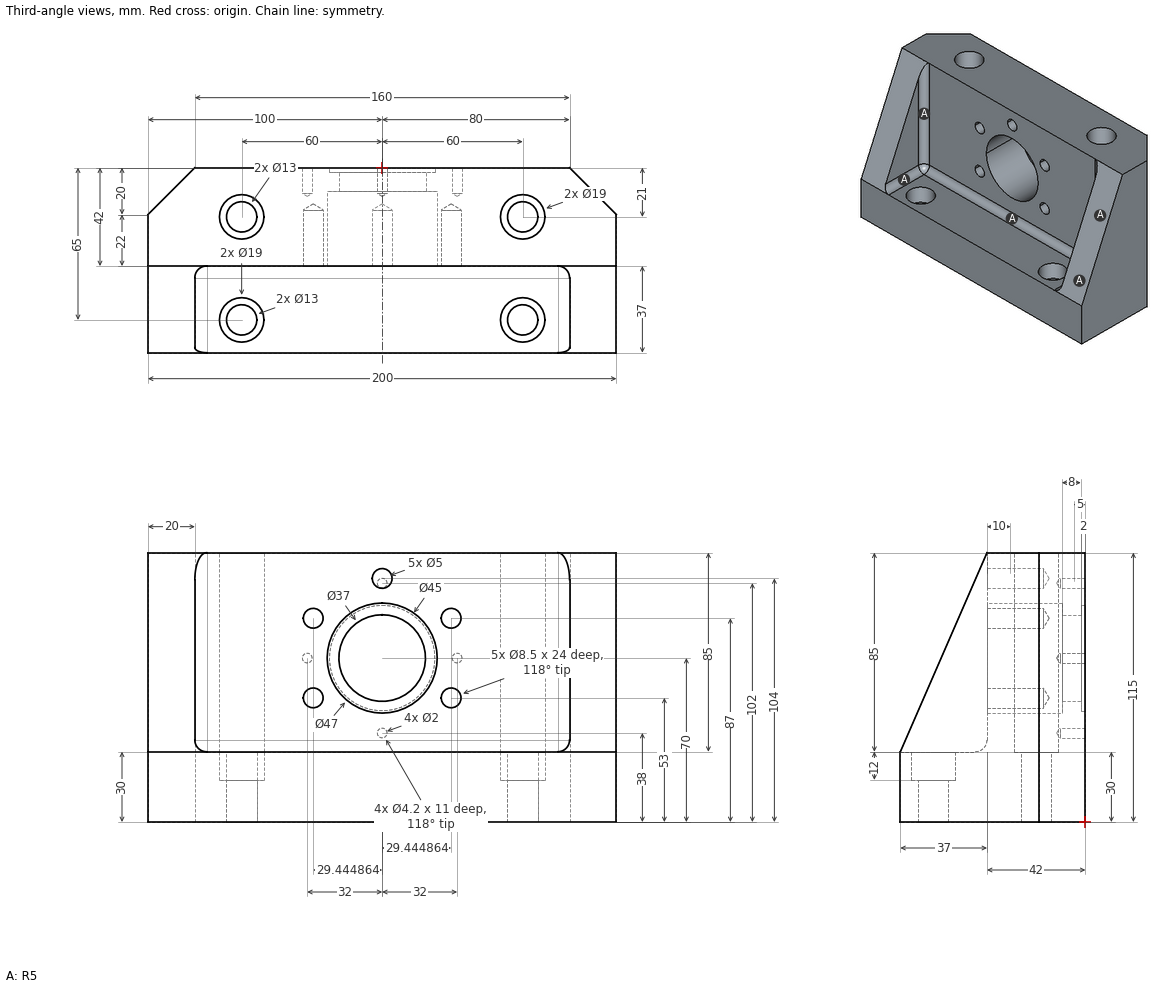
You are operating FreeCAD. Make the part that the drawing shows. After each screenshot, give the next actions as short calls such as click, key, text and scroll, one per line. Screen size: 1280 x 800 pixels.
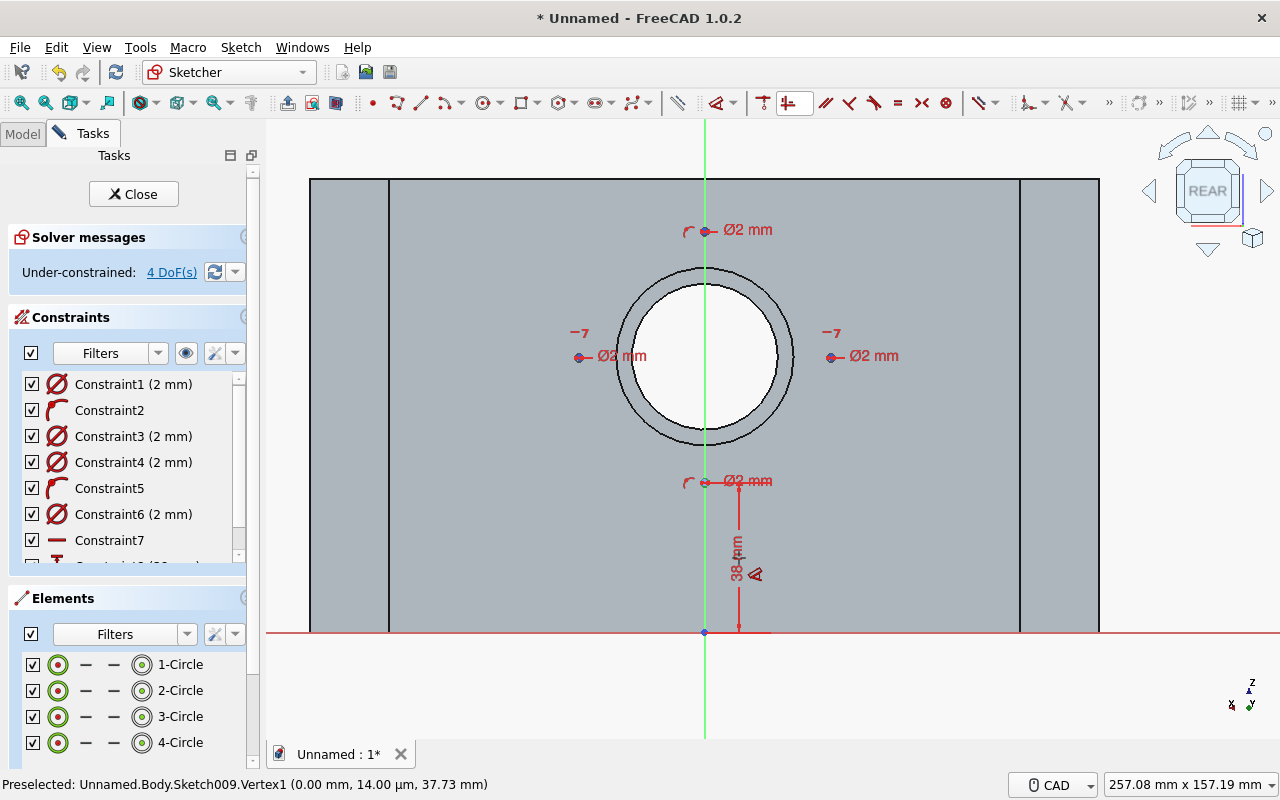
click(579, 358)
click(642, 667)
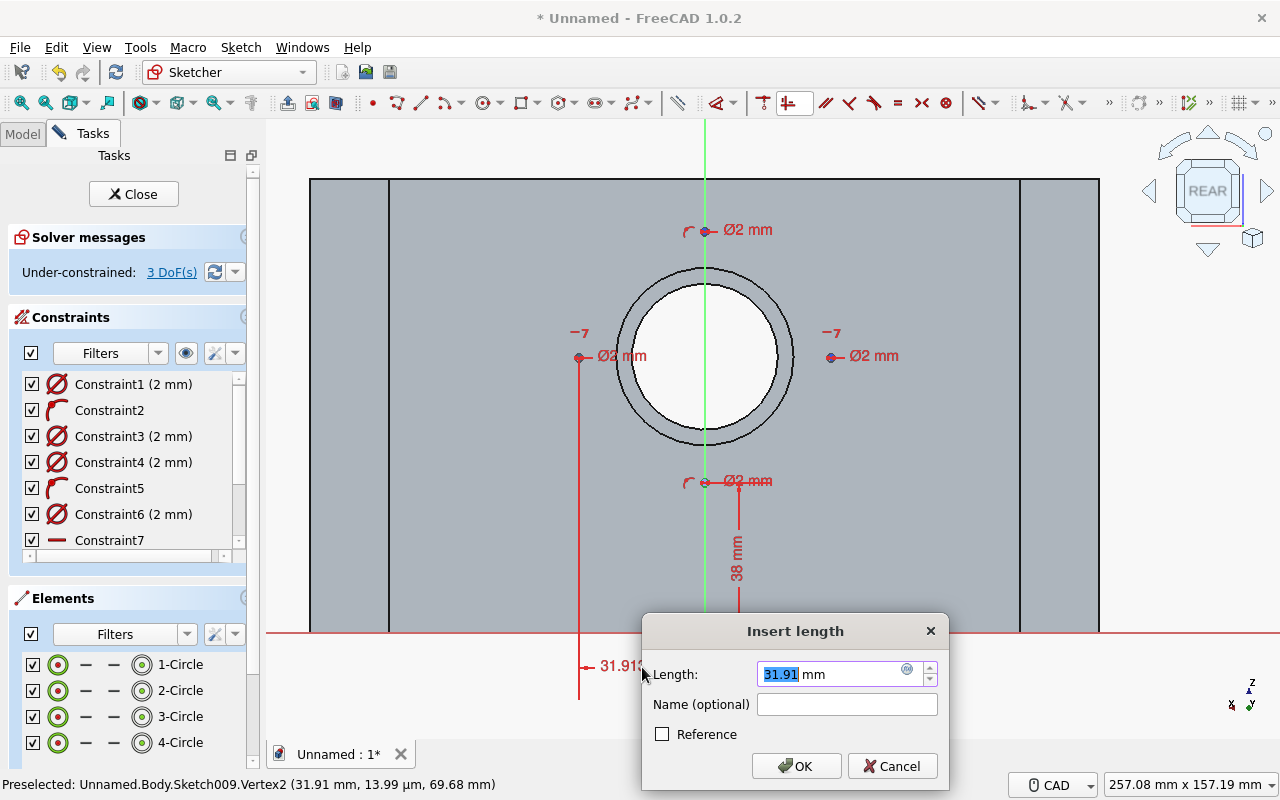
text(32)
key(Return)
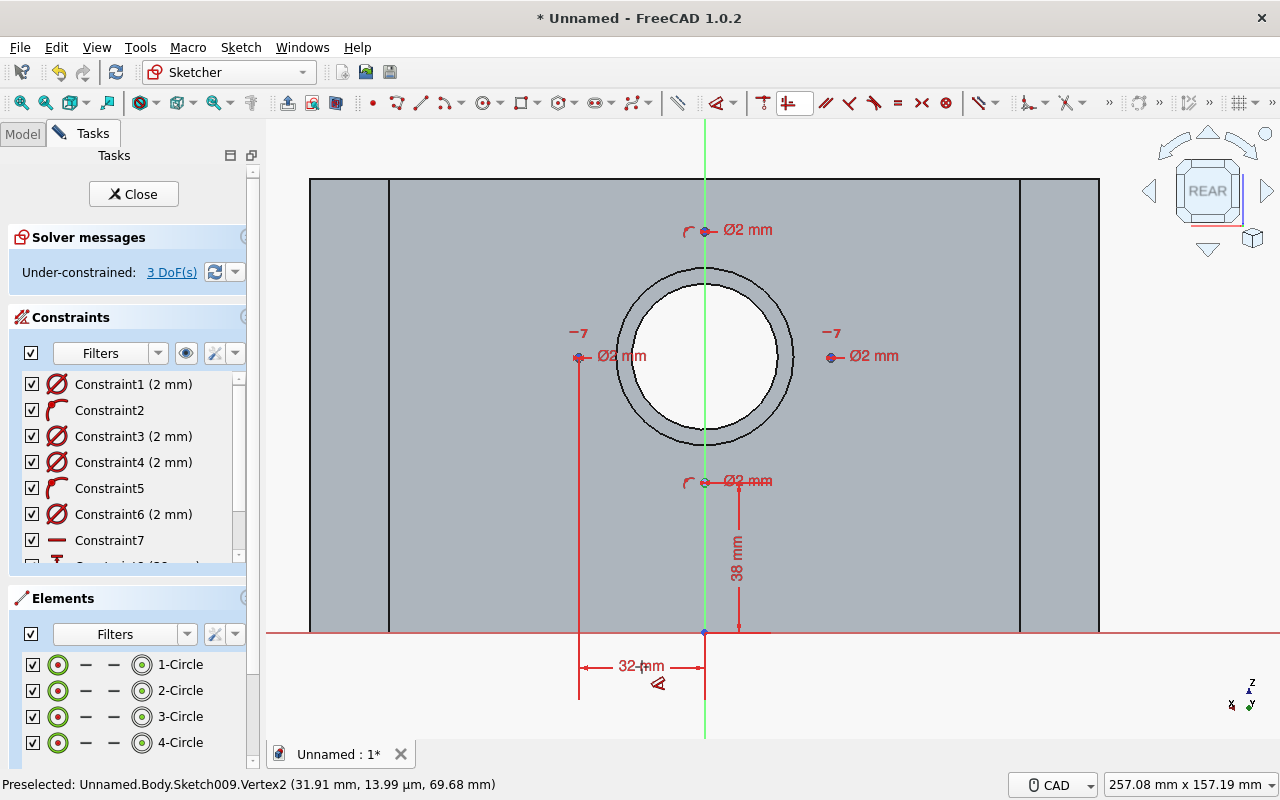
click(579, 358)
click(545, 495)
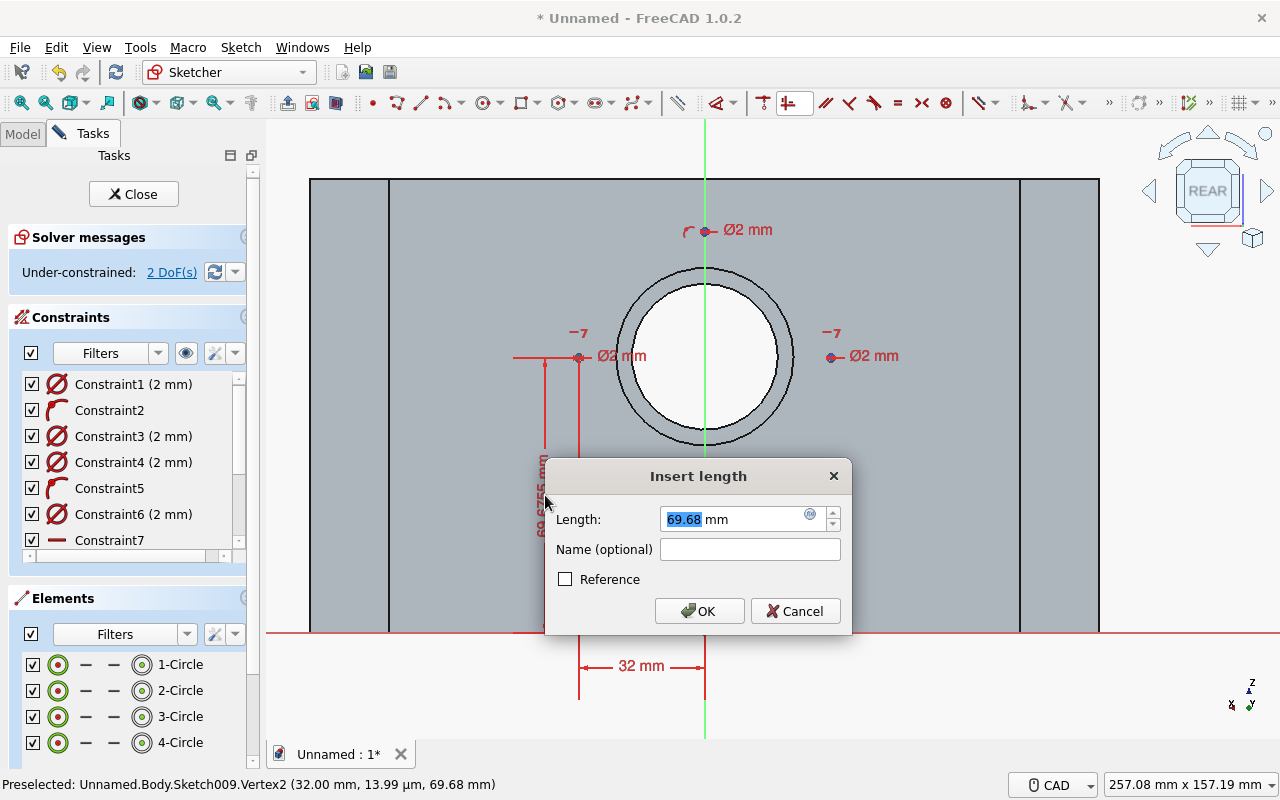
text(70)
key(Return)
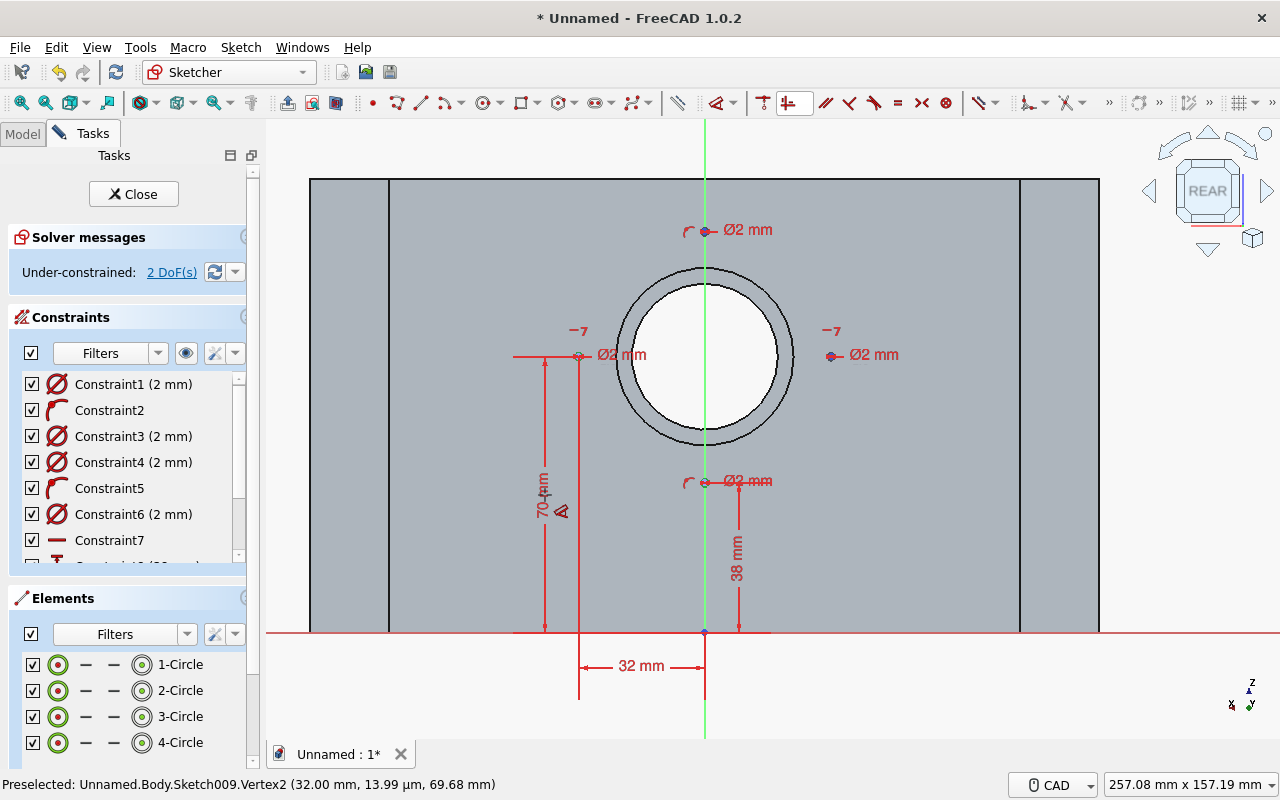
click(831, 357)
click(768, 667)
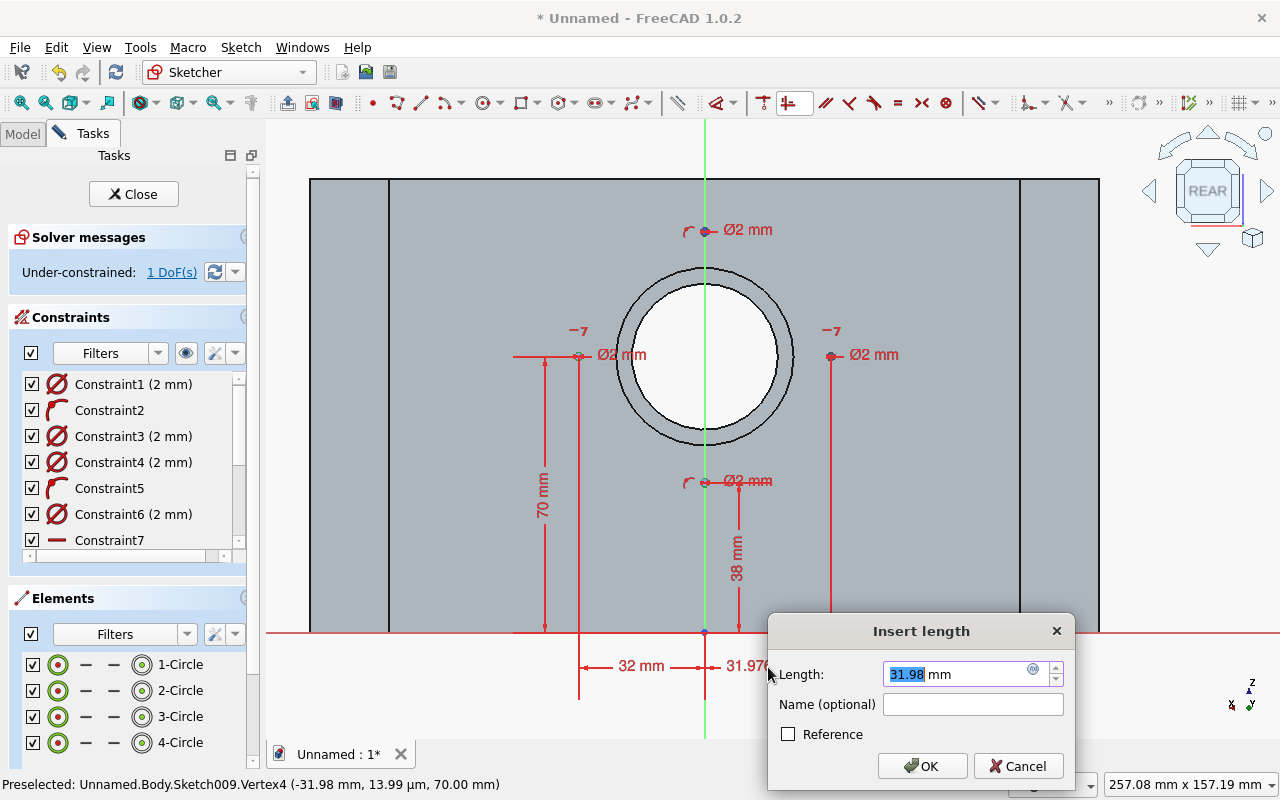
text(32)
key(Return)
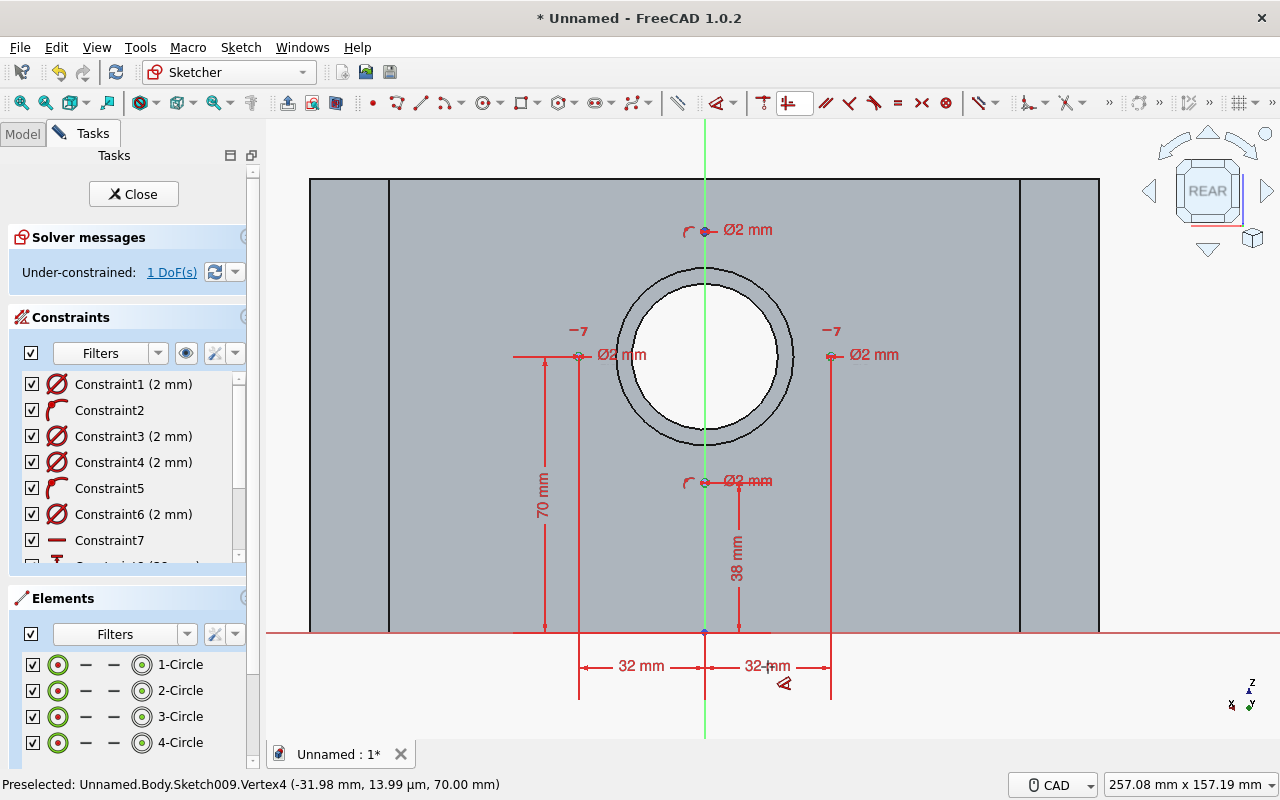
click(705, 232)
click(739, 432)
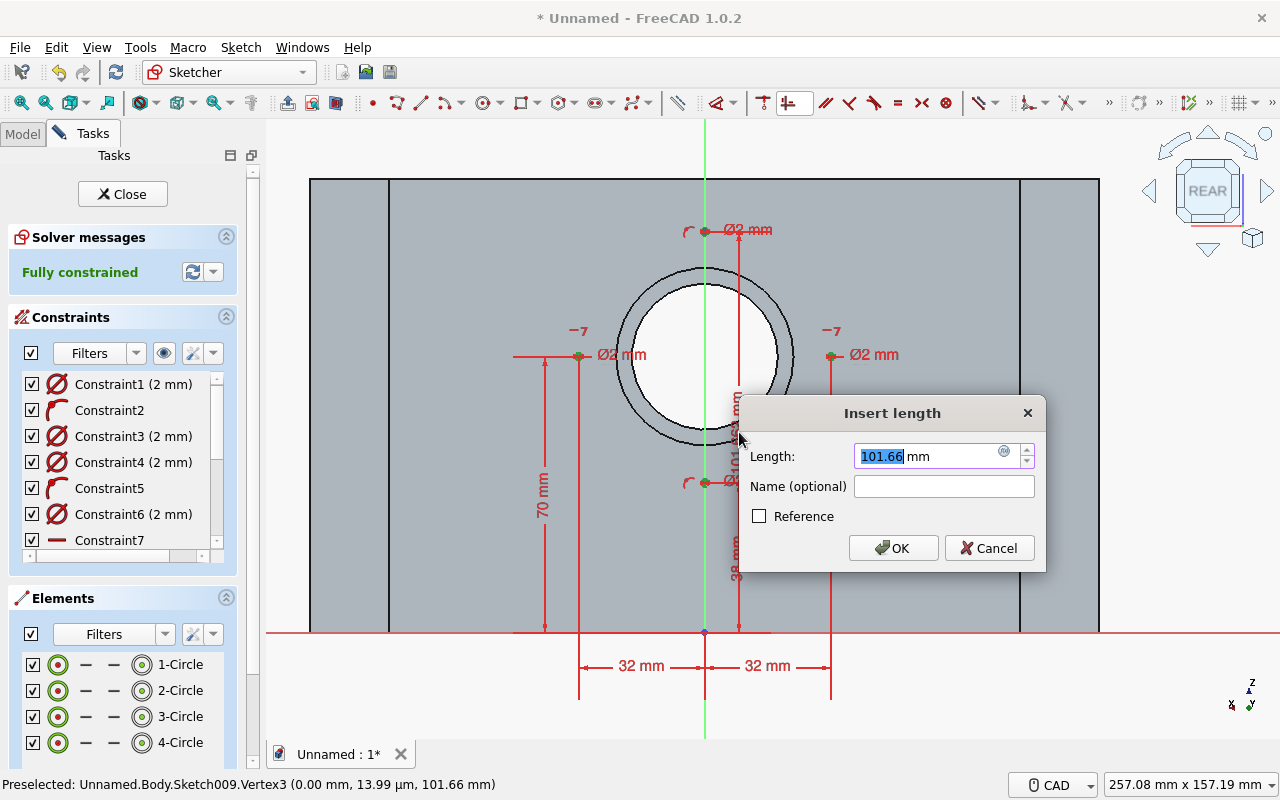
text(102)
key(Return)
key(Escape)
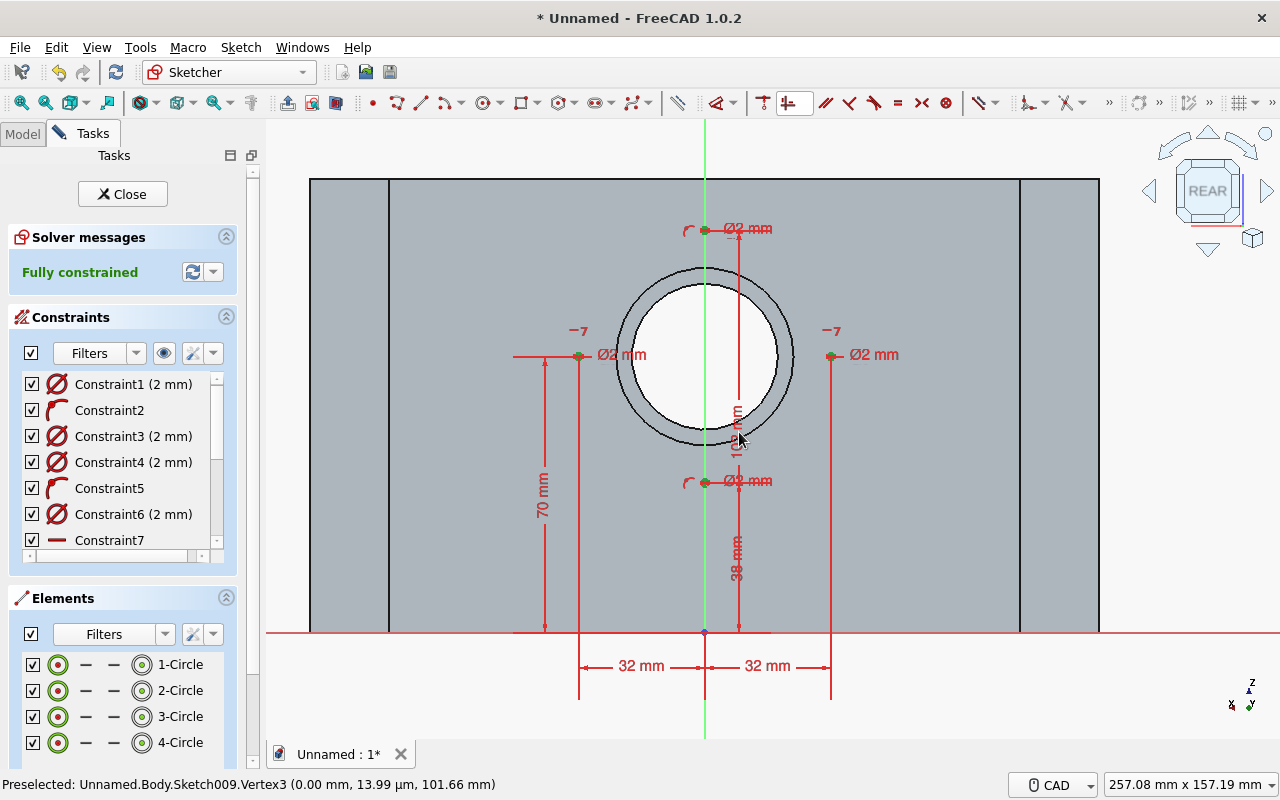
click(123, 194)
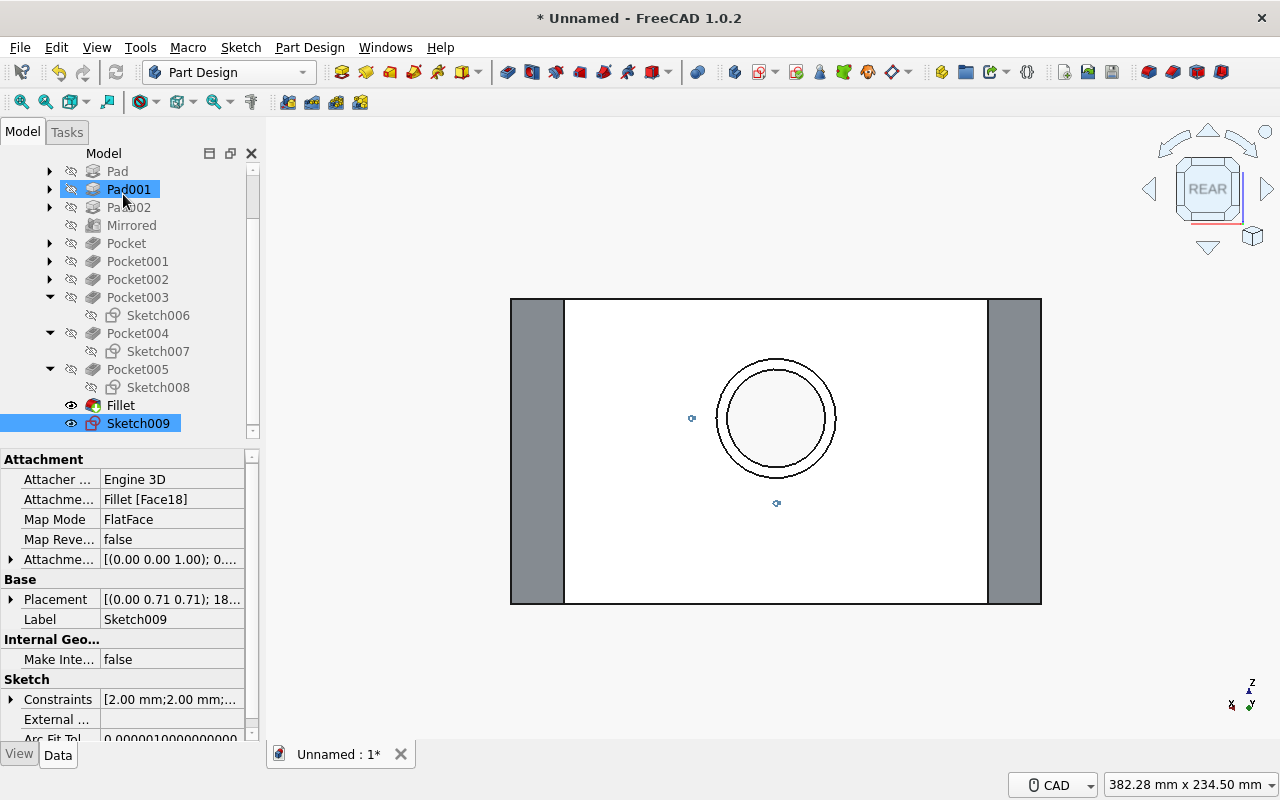
click(508, 72)